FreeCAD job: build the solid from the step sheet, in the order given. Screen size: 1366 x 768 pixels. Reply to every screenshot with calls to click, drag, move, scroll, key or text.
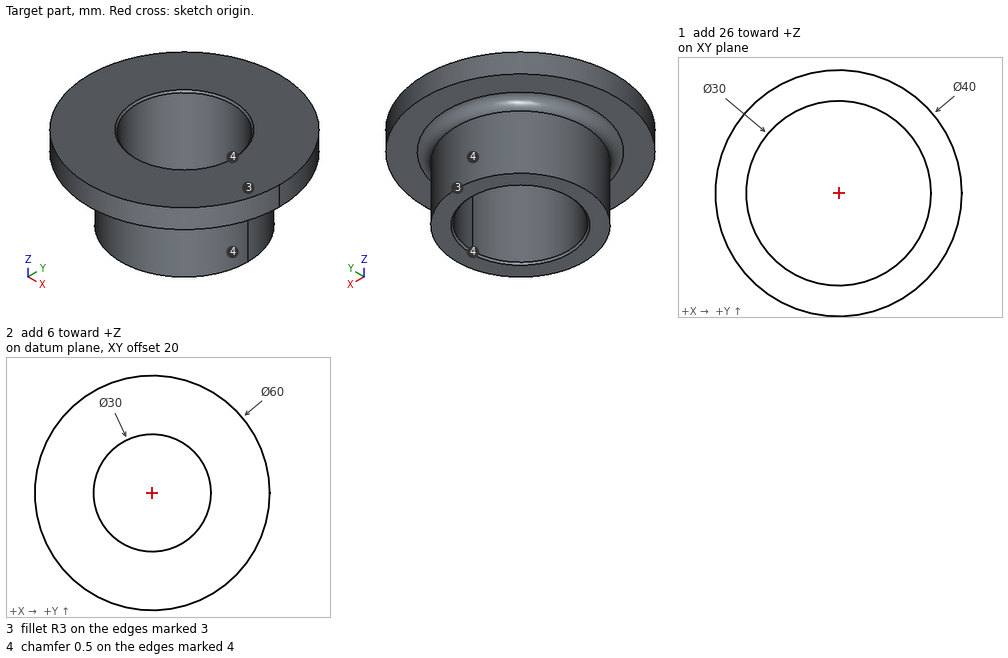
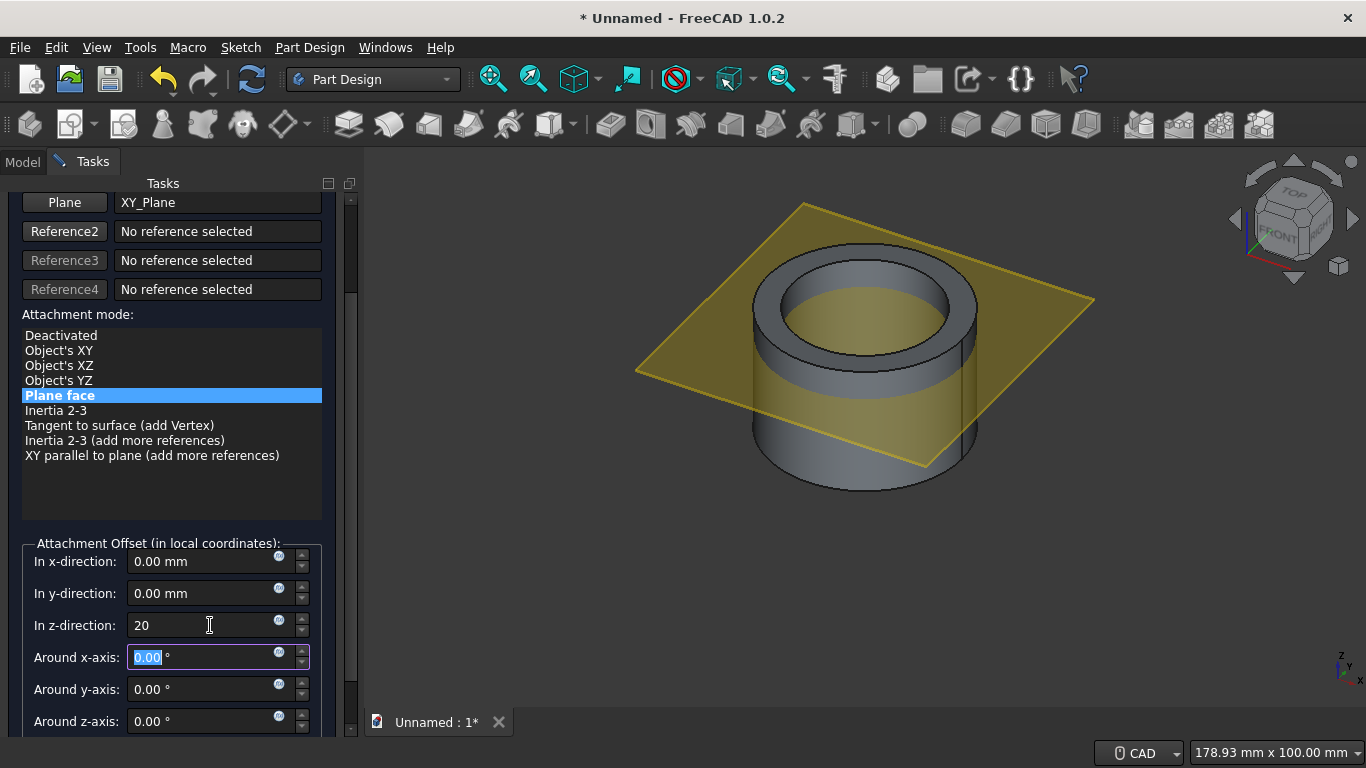
scroll(351, 464, up, 3)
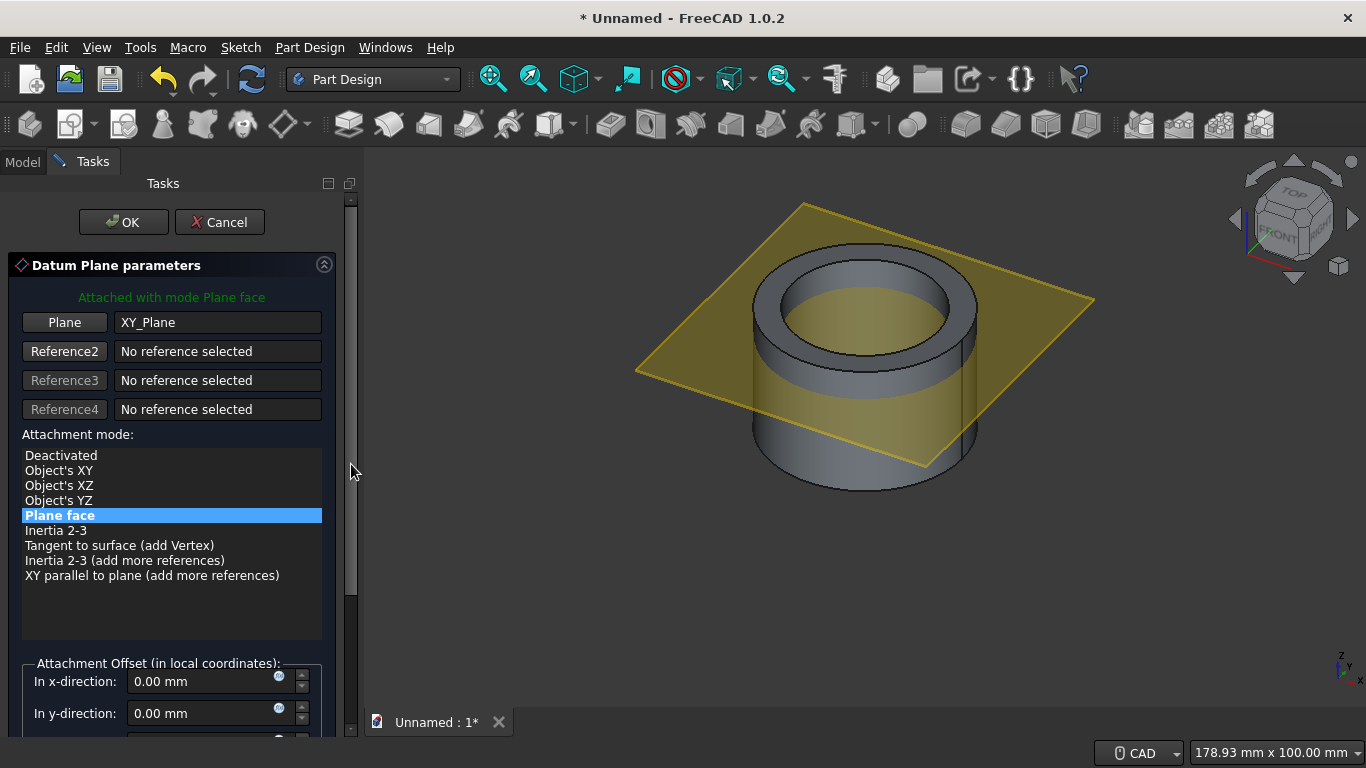
click(124, 222)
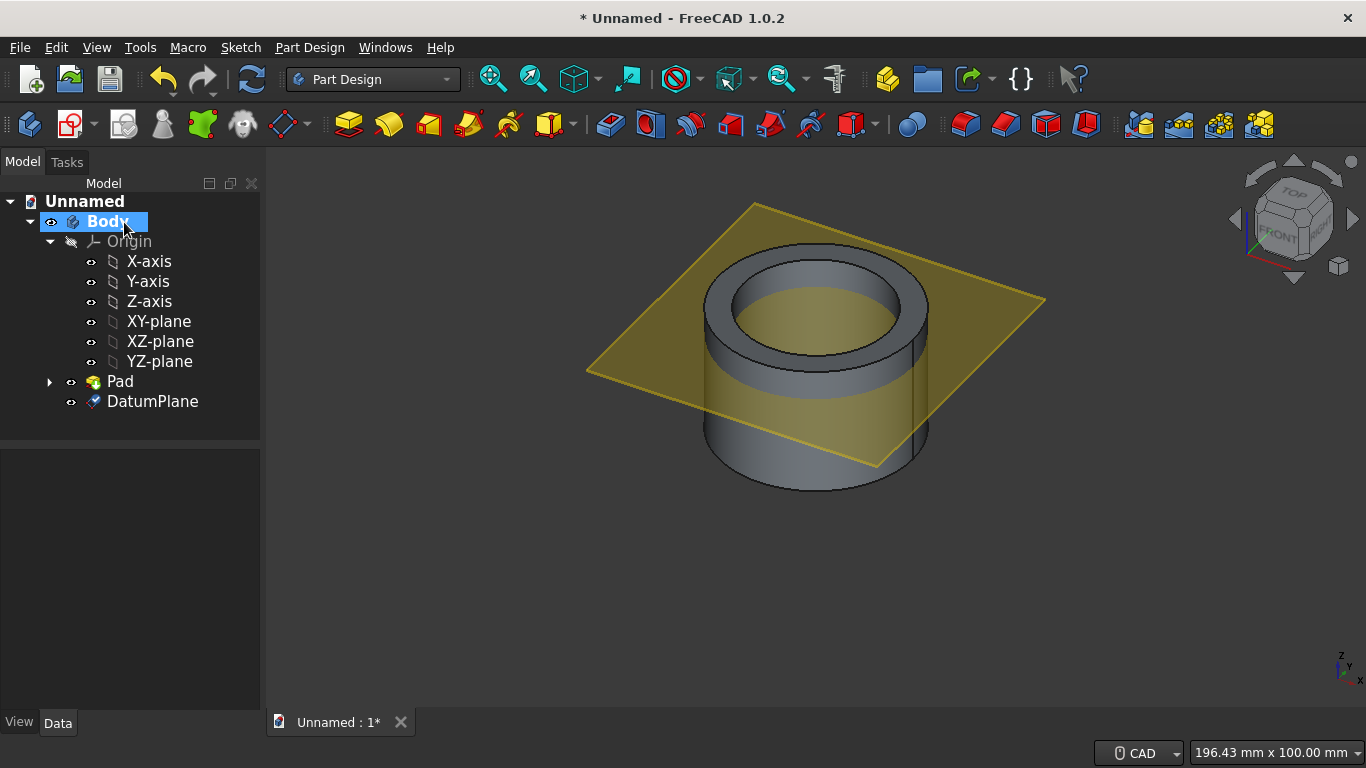
click(116, 402)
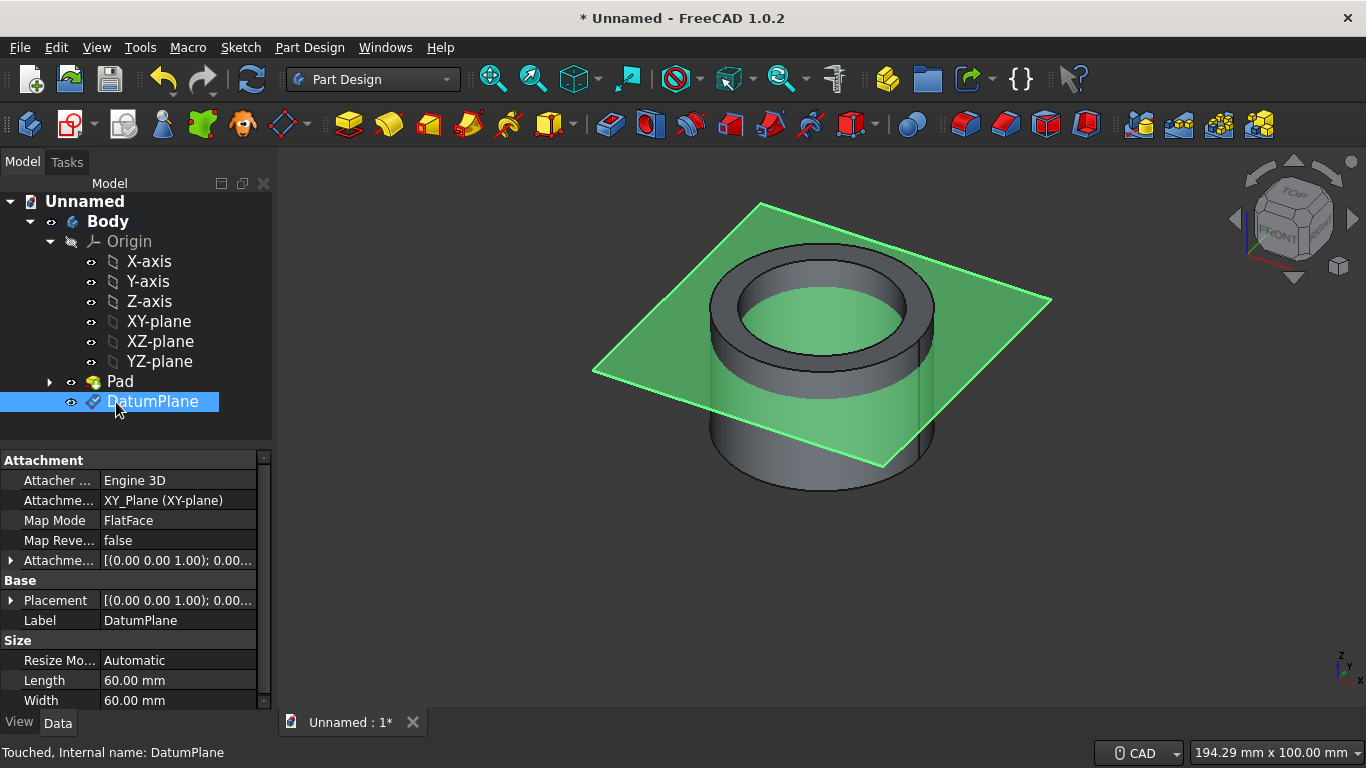
click(70, 124)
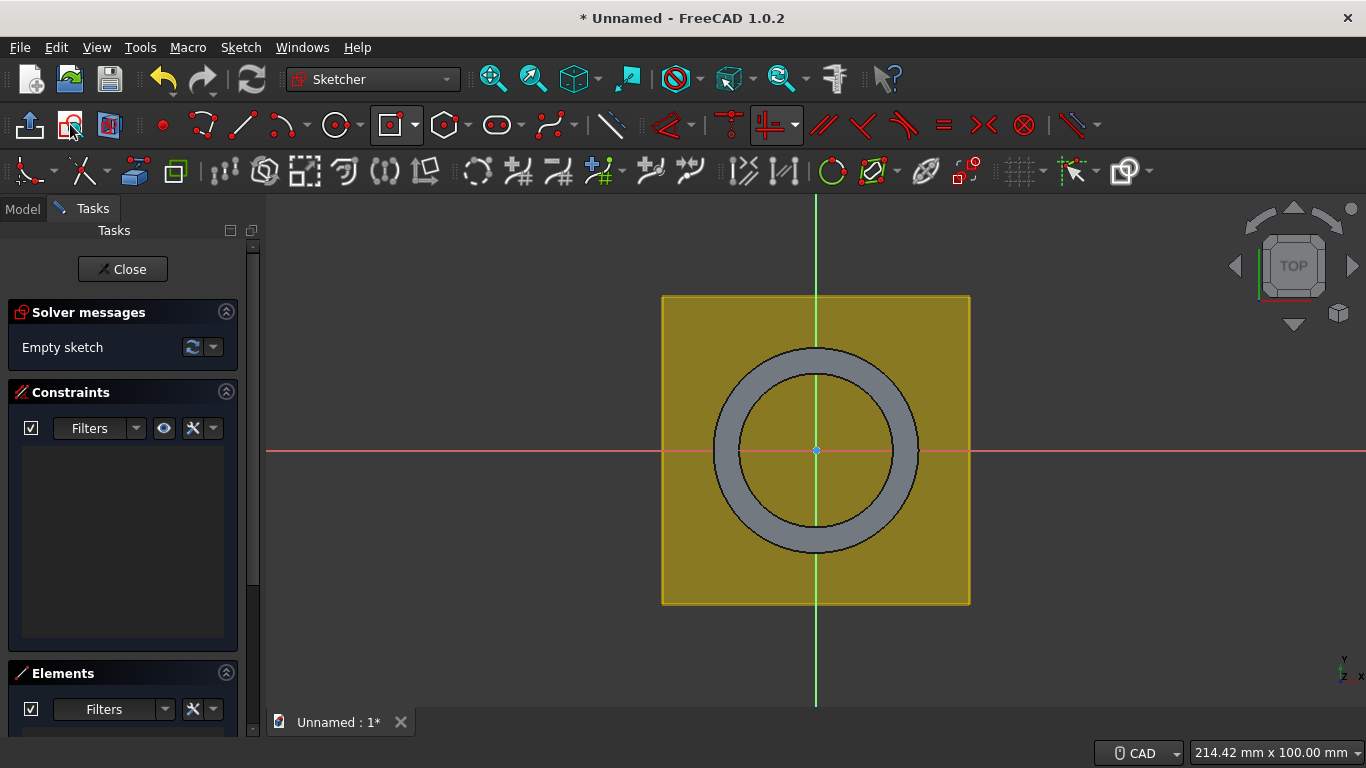
click(110, 126)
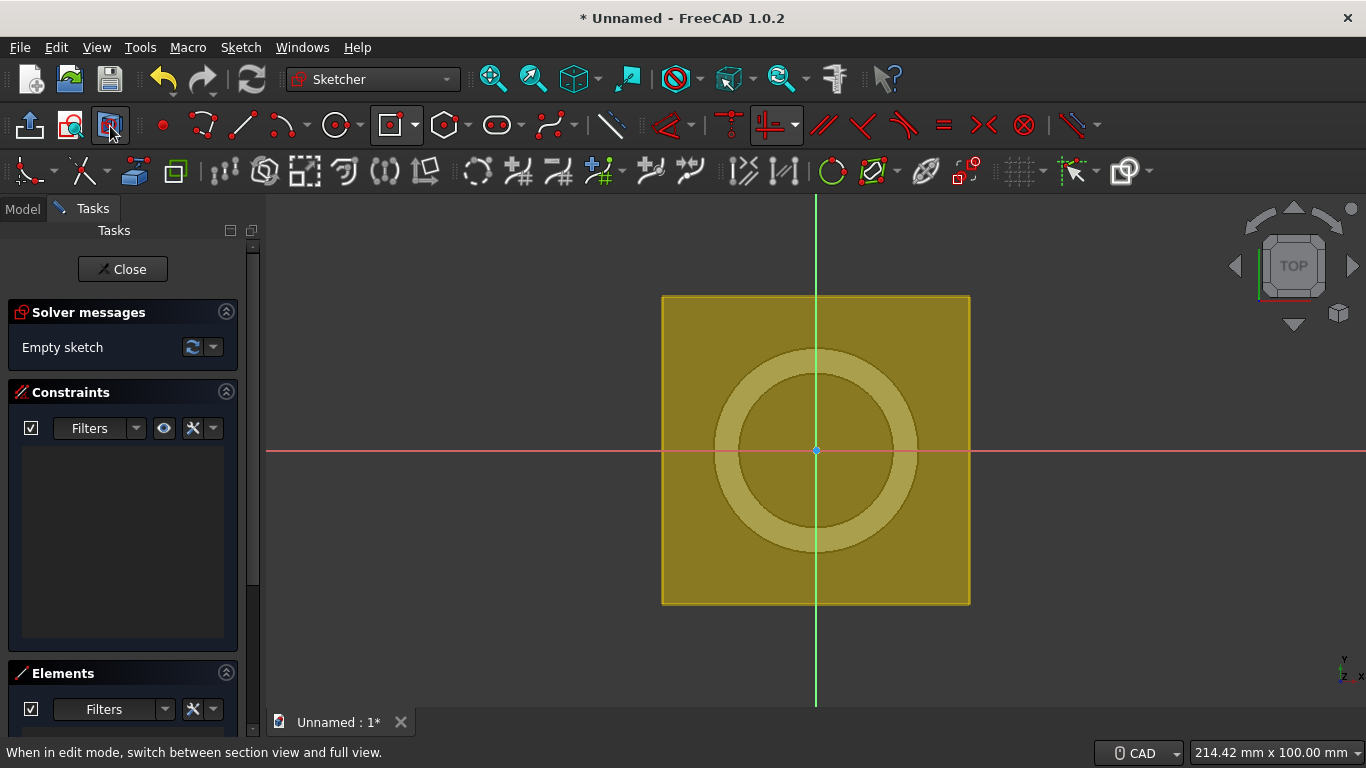
click(336, 126)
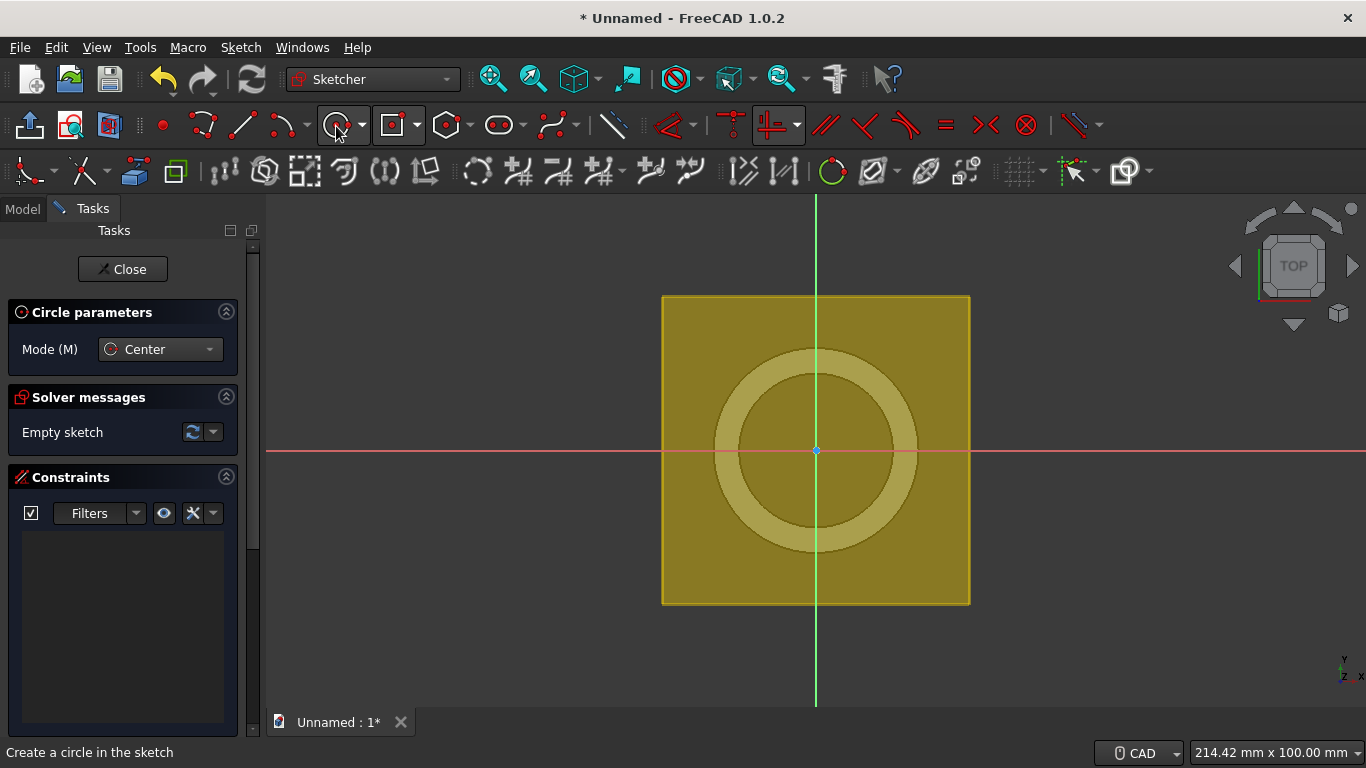
click(816, 450)
move(925, 342)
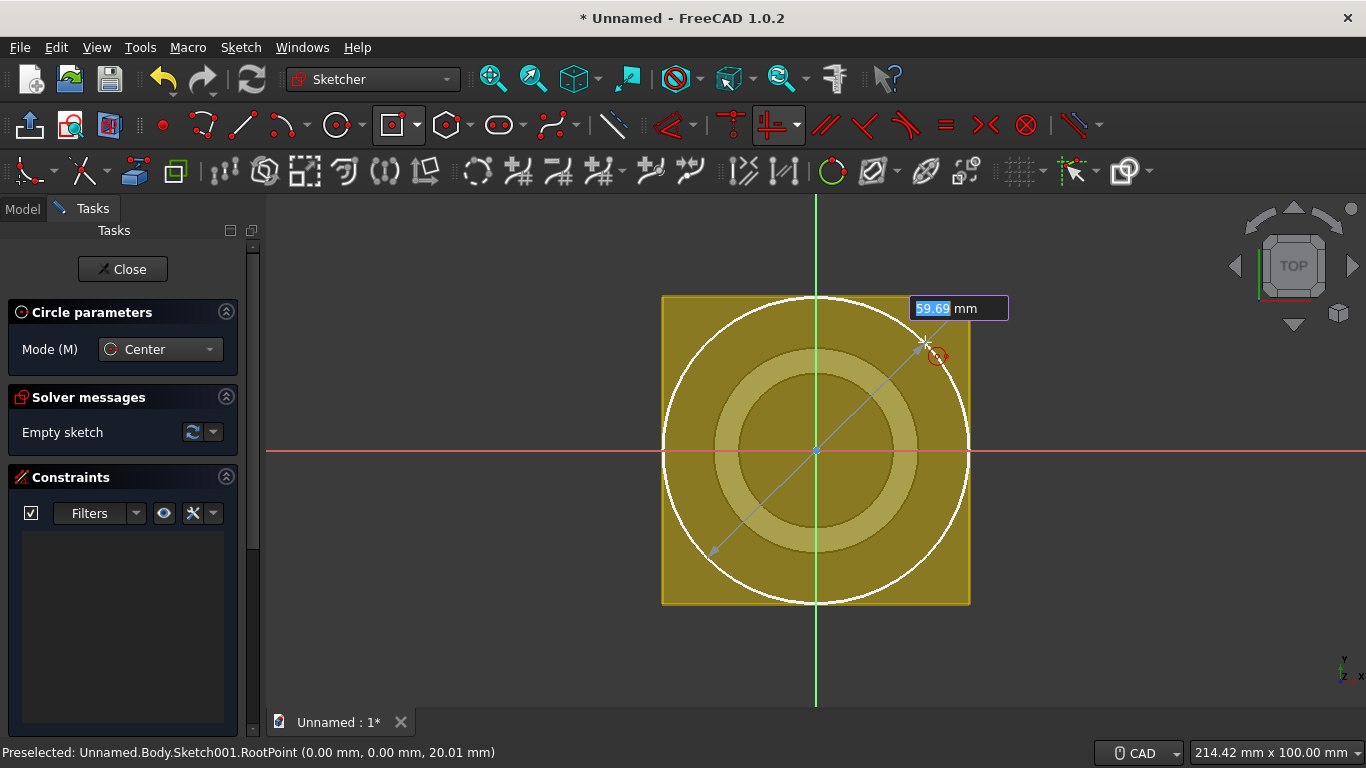
text(60)
key(Return)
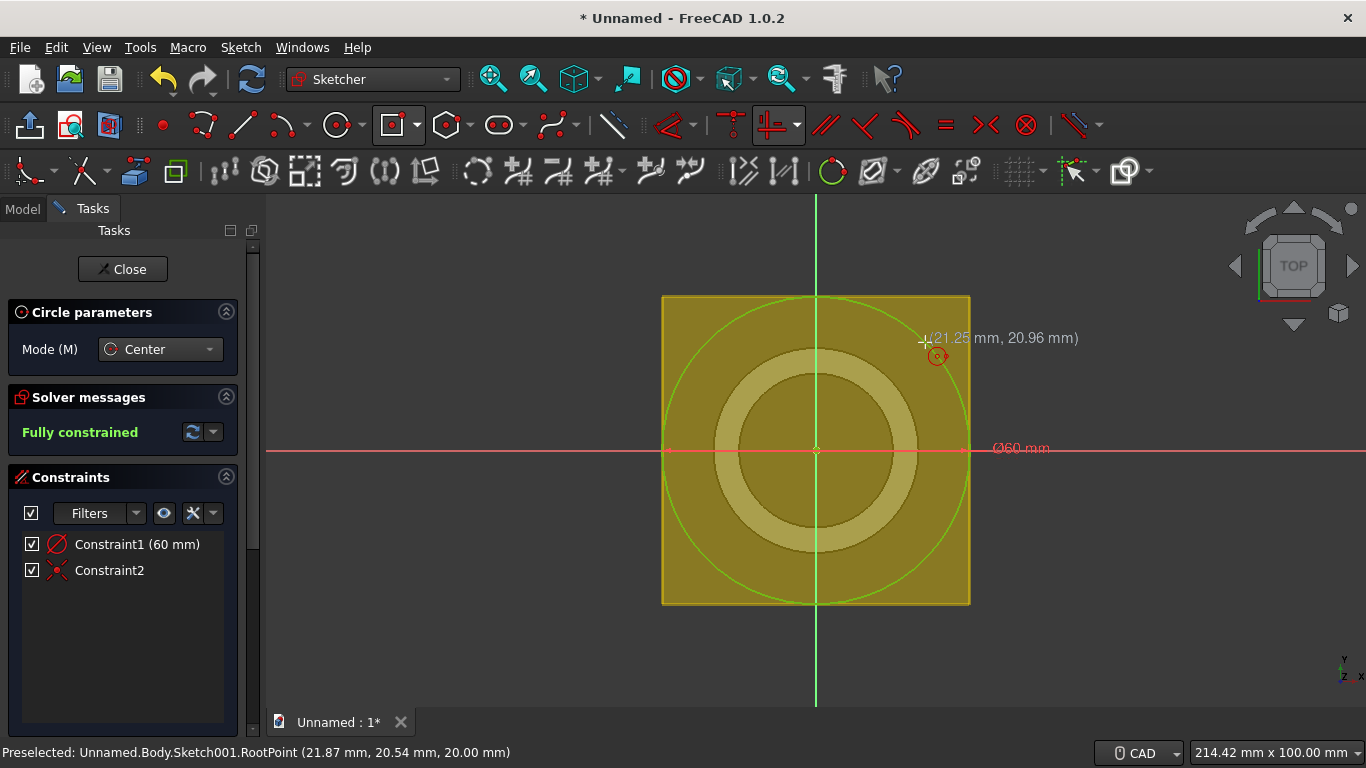
click(816, 450)
move(870, 396)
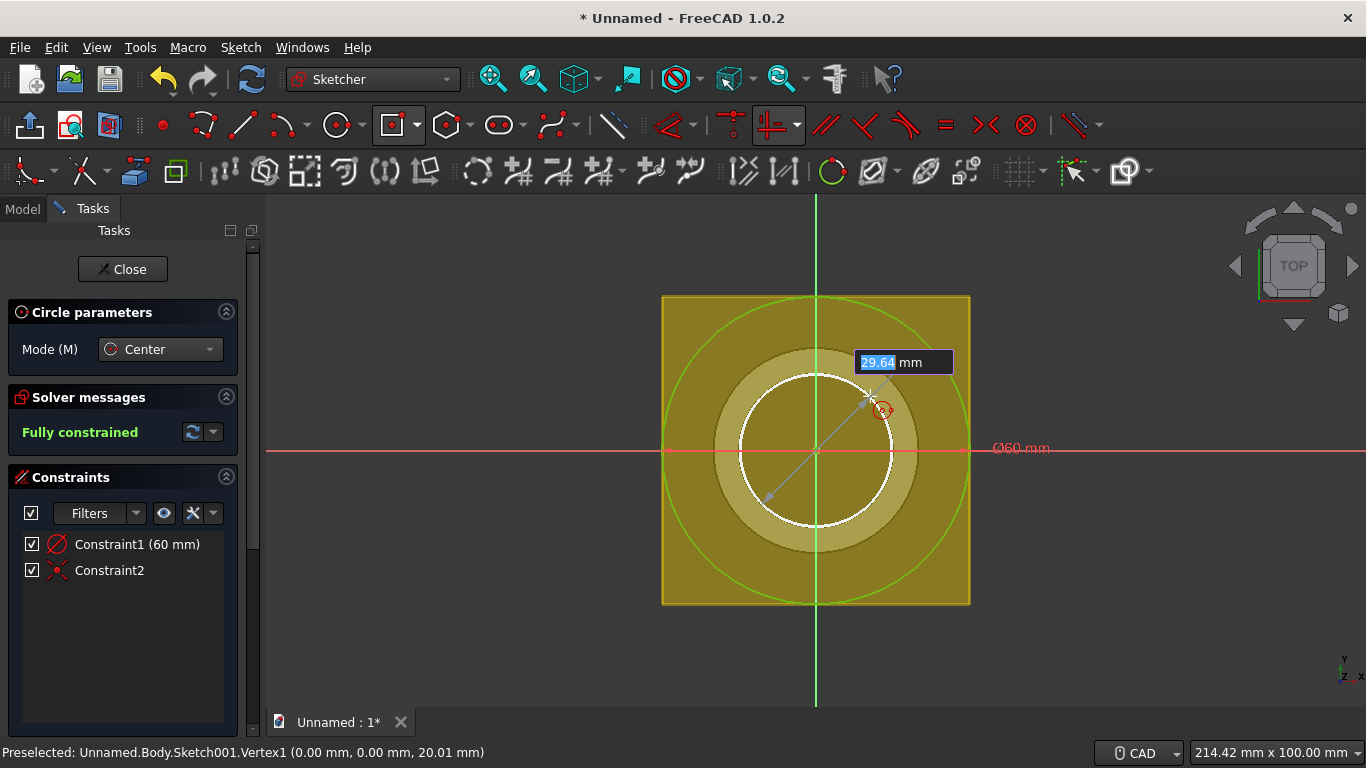
text(30)
key(Return)
key(Escape)